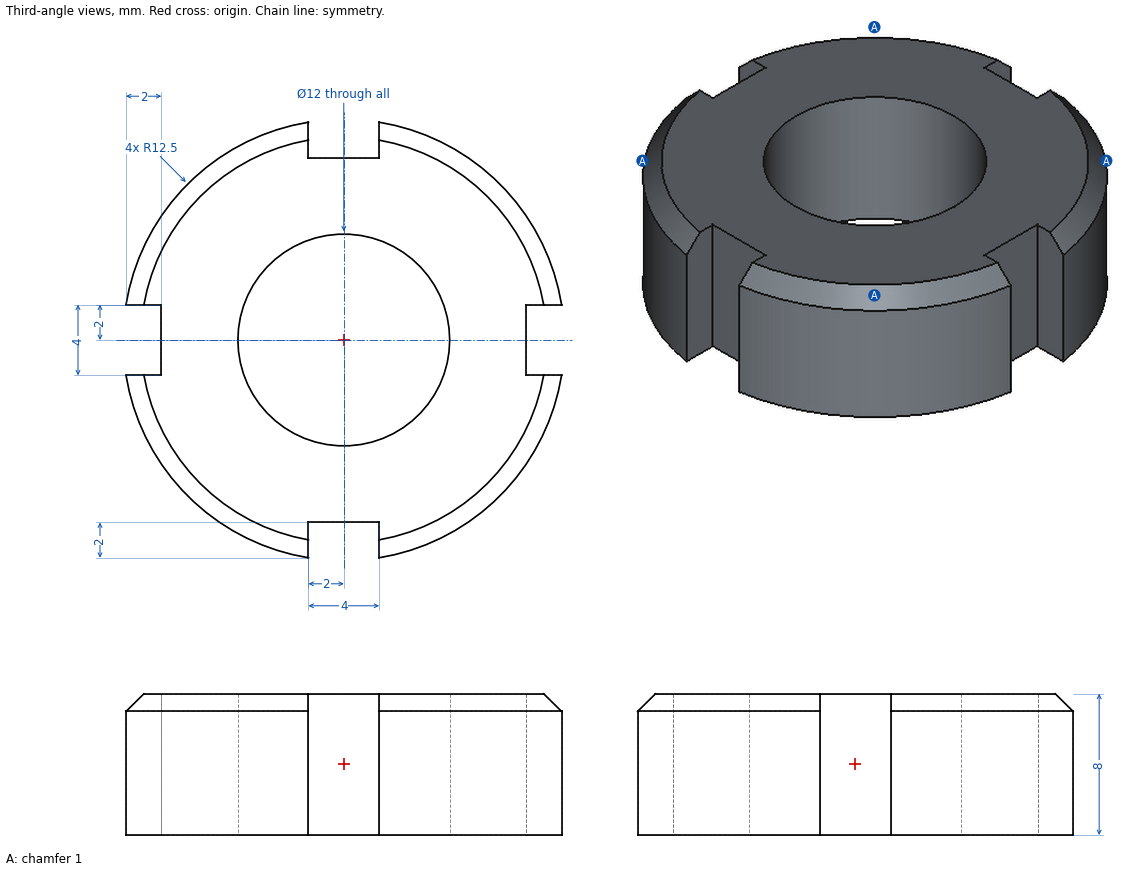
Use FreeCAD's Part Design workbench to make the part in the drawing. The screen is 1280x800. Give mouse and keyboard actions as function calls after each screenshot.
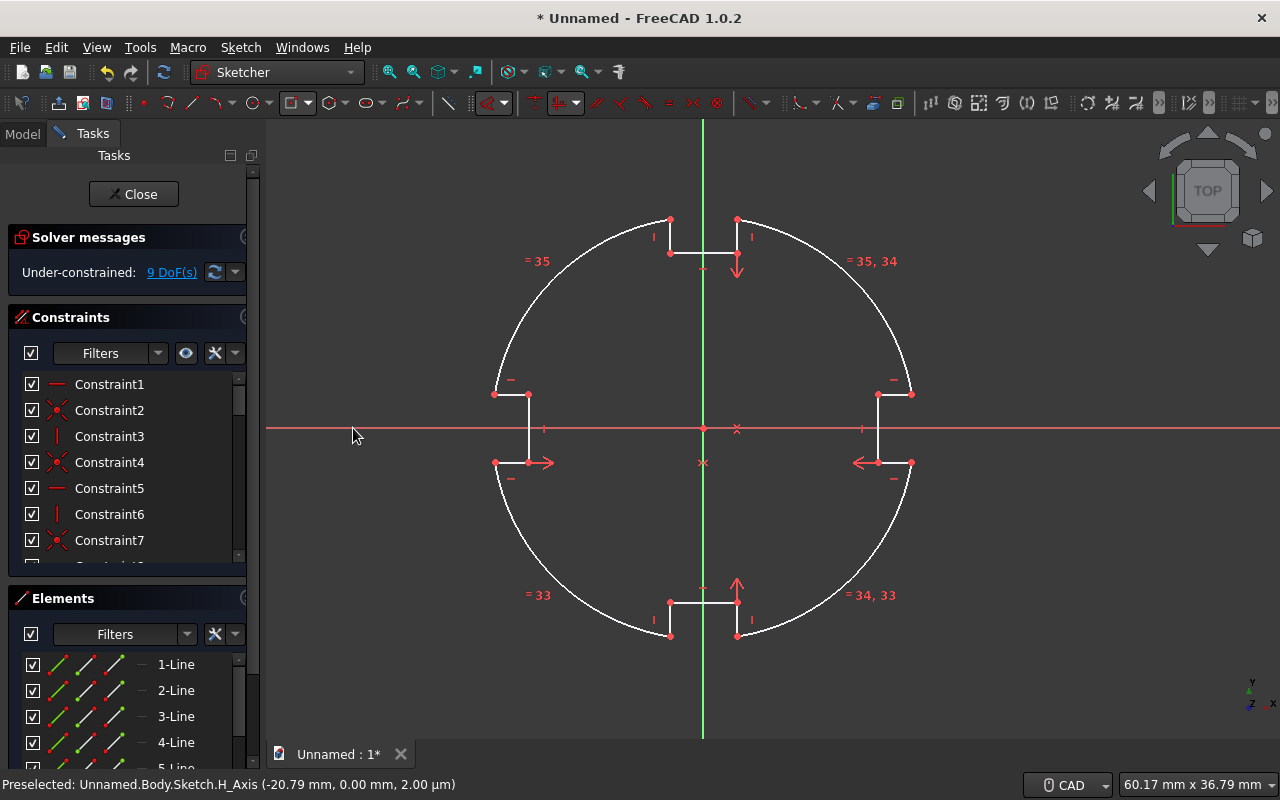
click(522, 537)
click(495, 553)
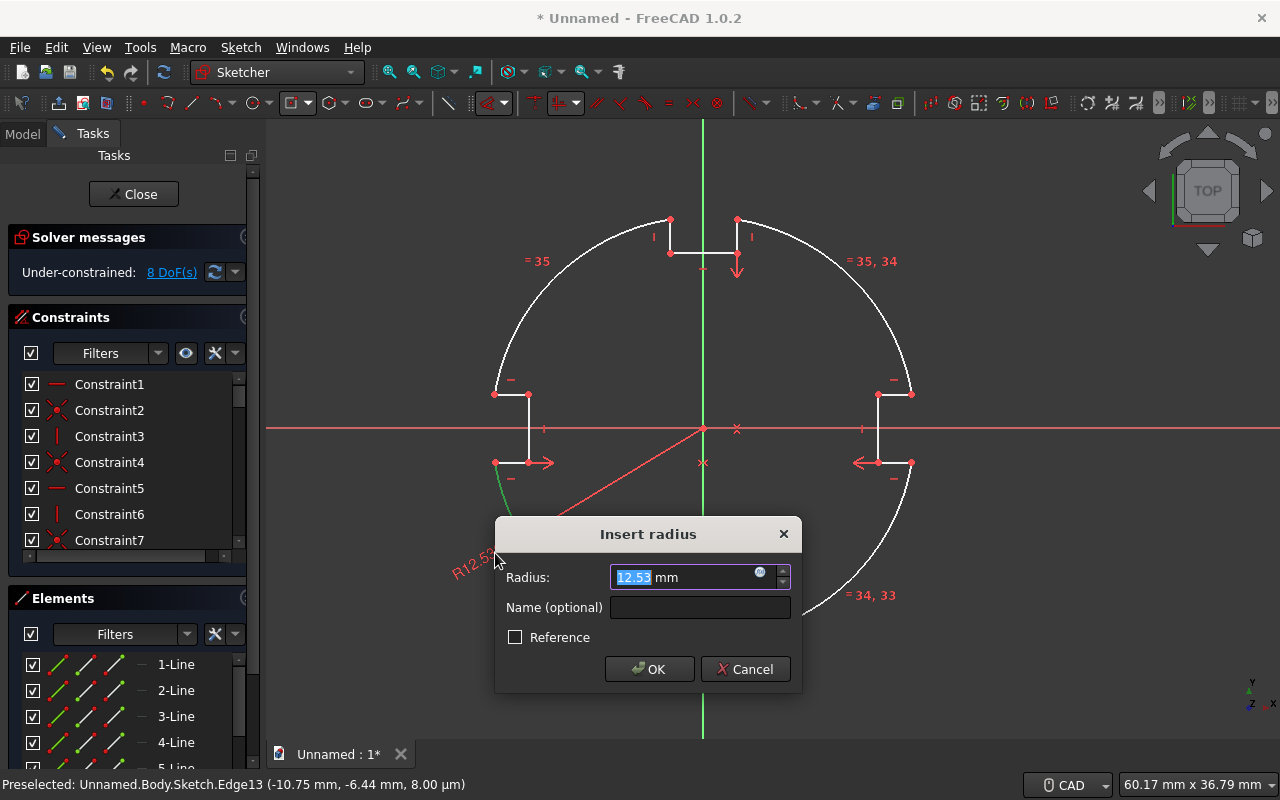
text(12.5)
key(Return)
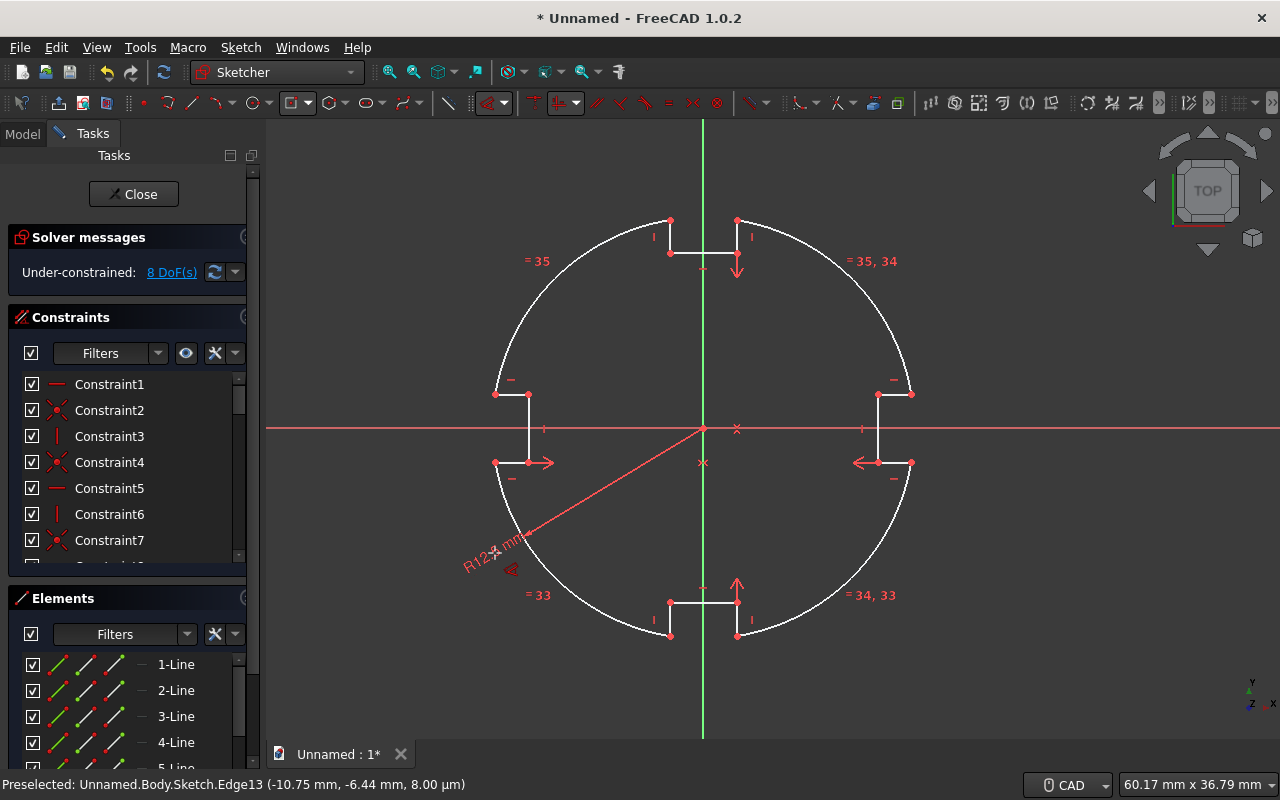
scroll(505, 395, up, 2)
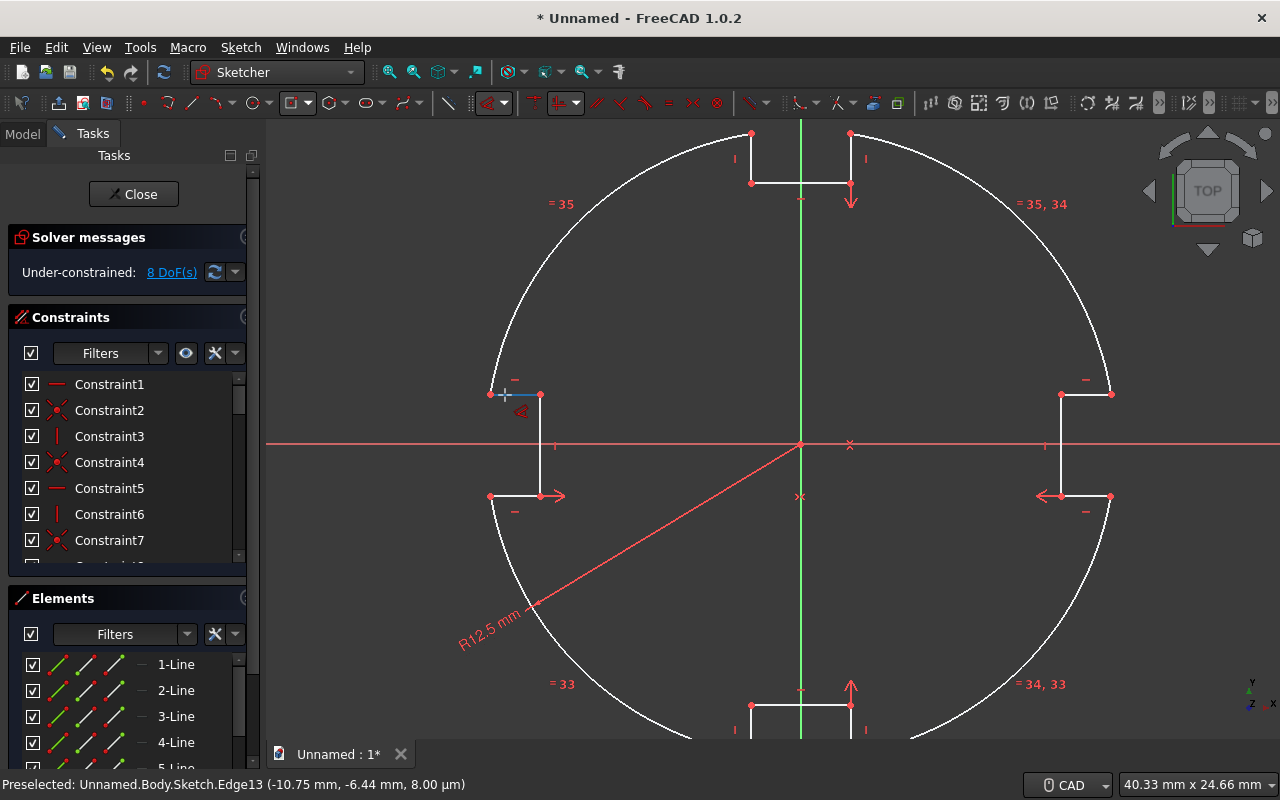
click(505, 395)
click(515, 361)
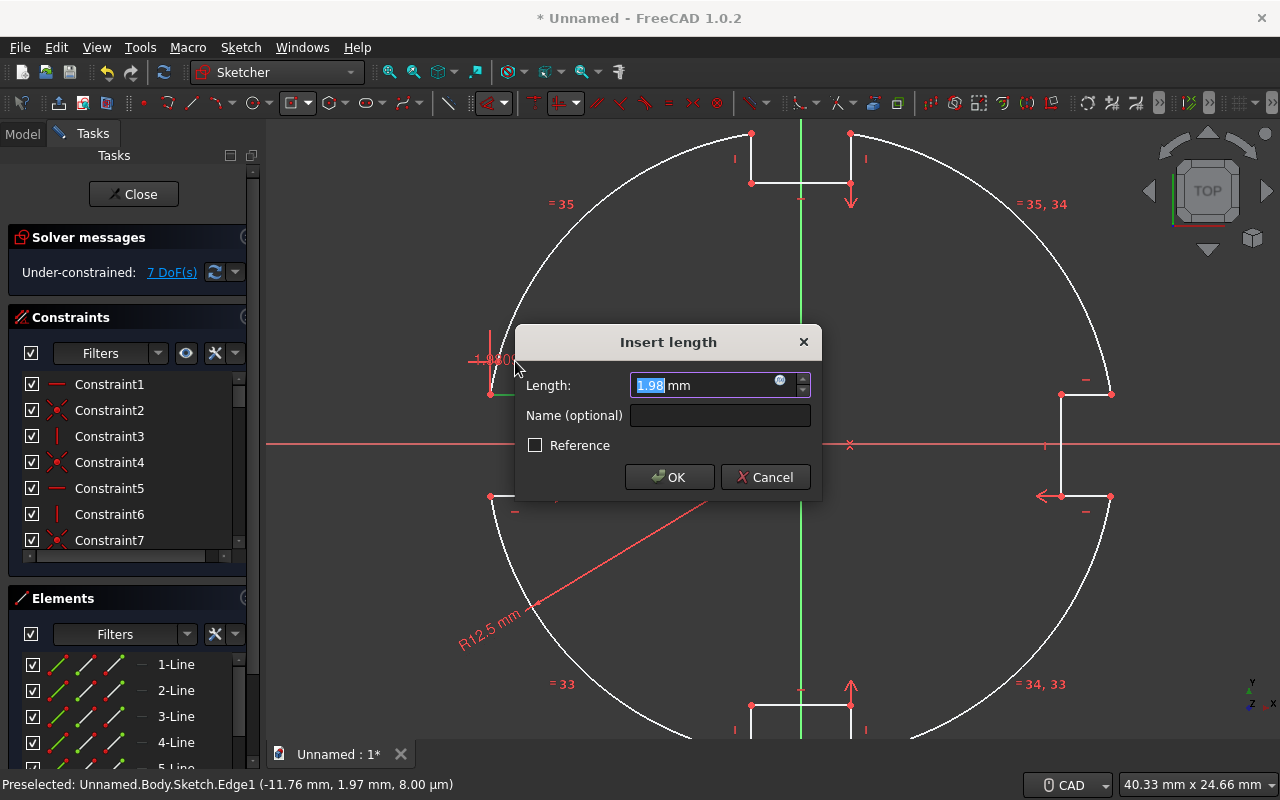
text(2)
key(Return)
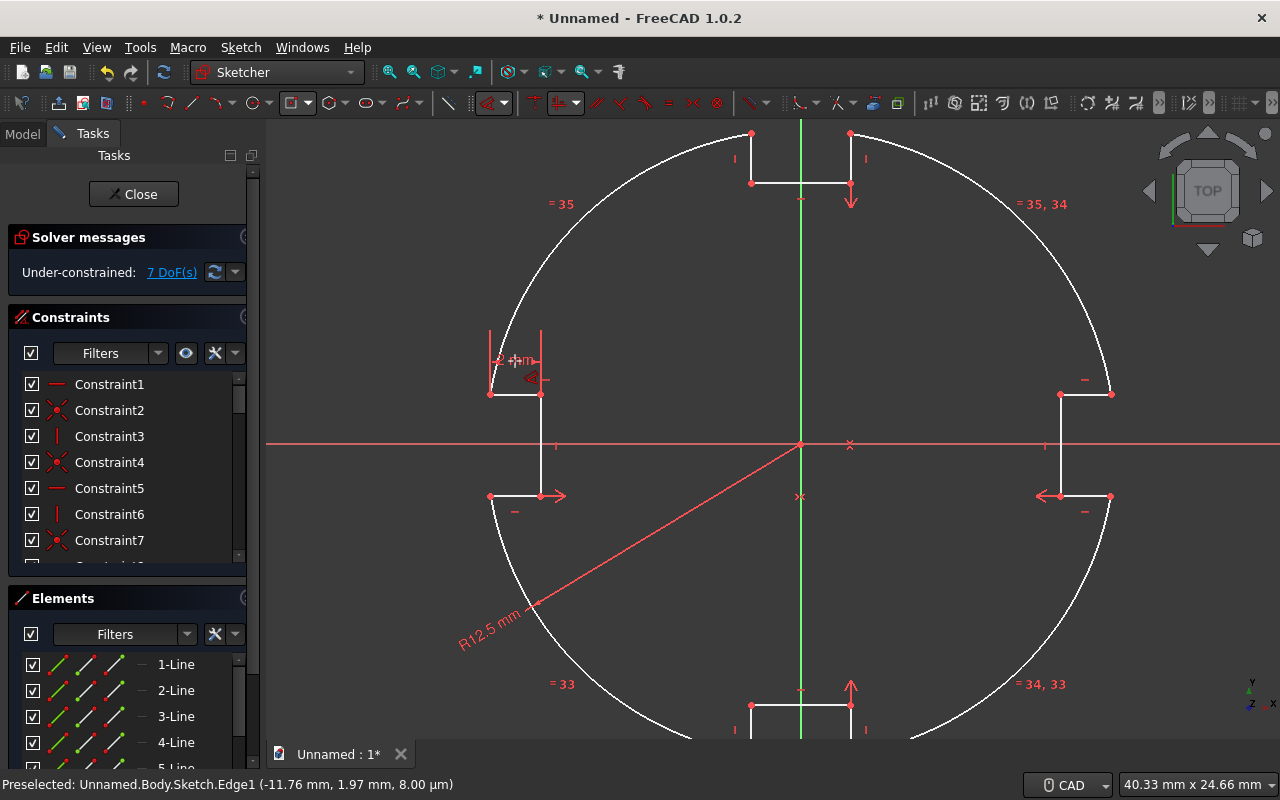
click(541, 425)
click(507, 422)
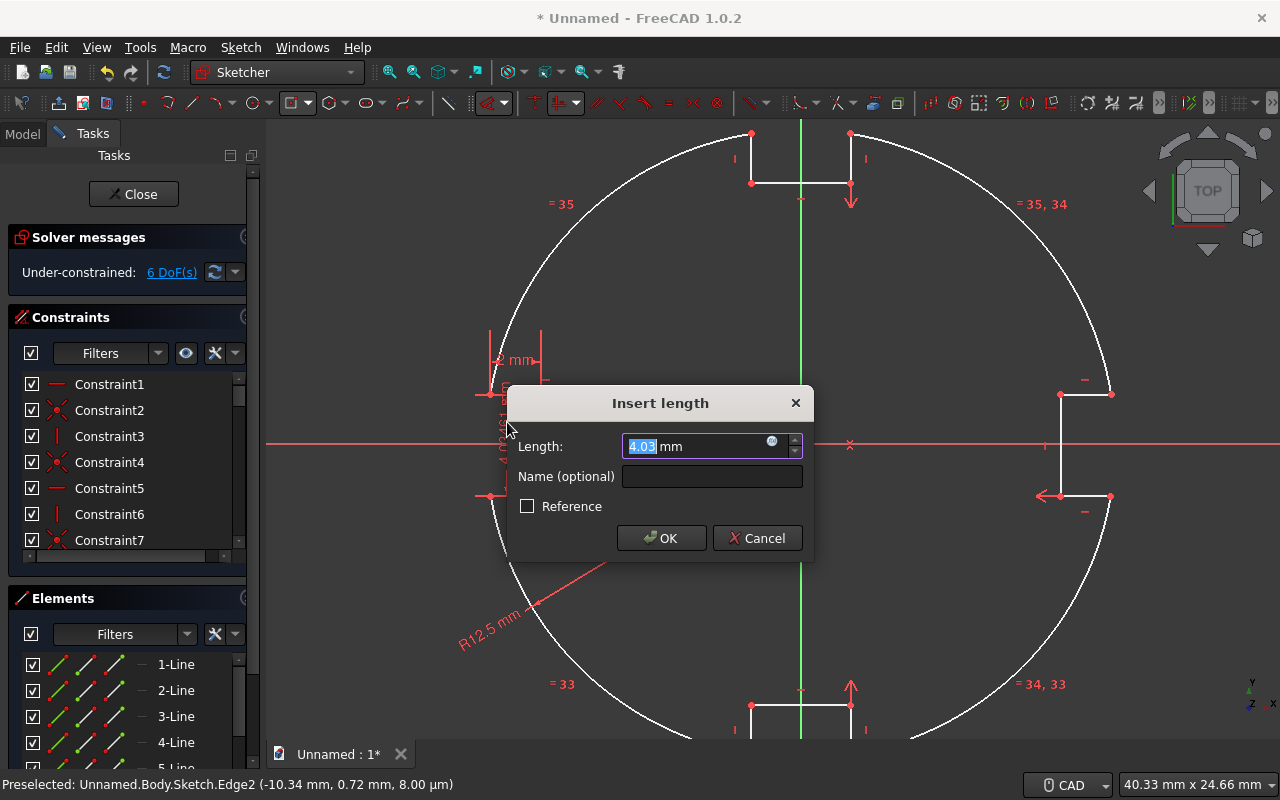
text(4)
key(Return)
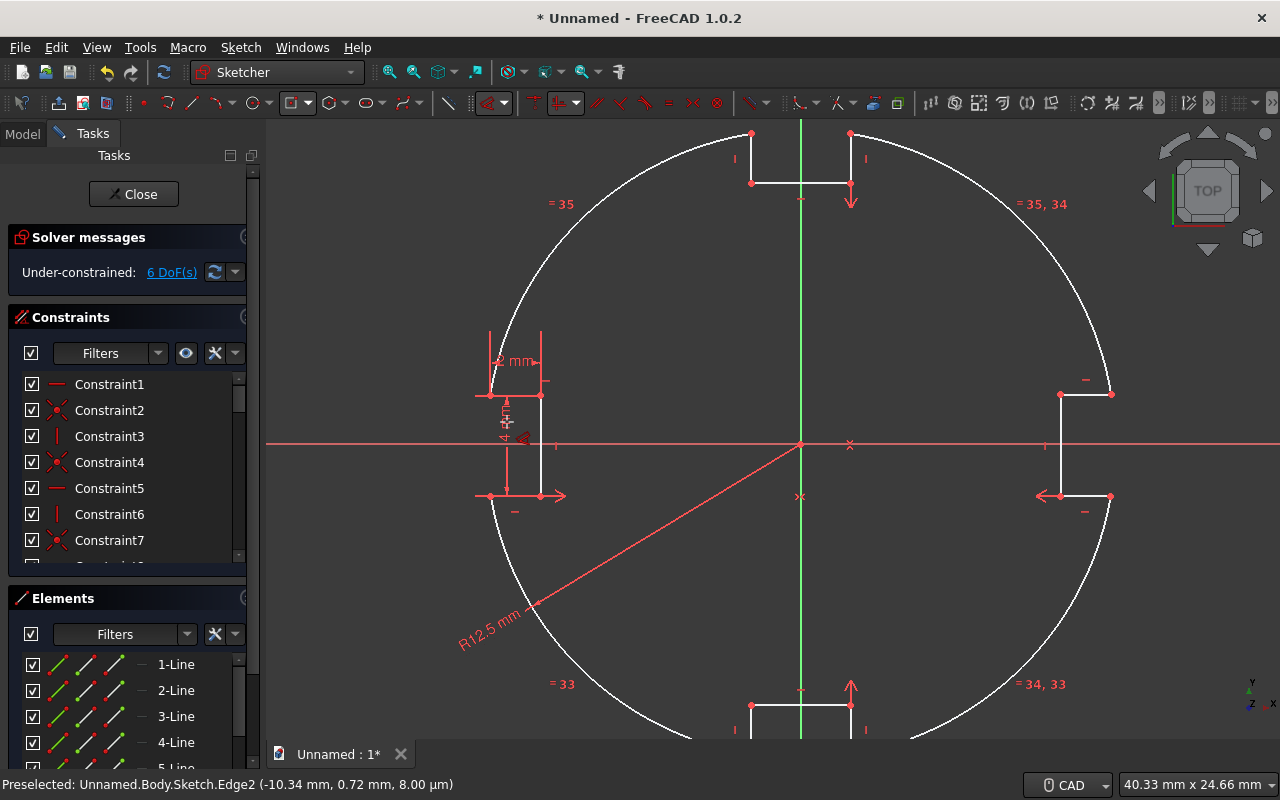
scroll(509, 398, down, 2)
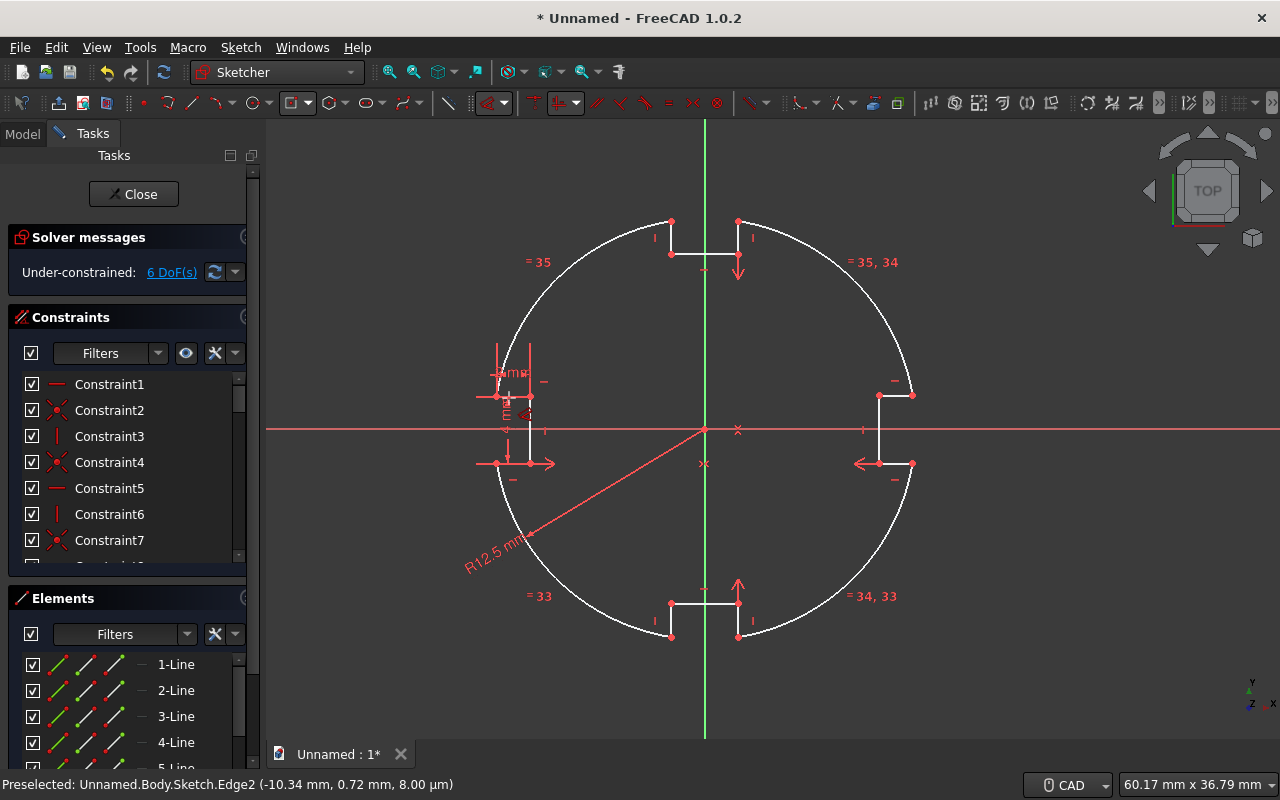
scroll(671, 627, up, 2)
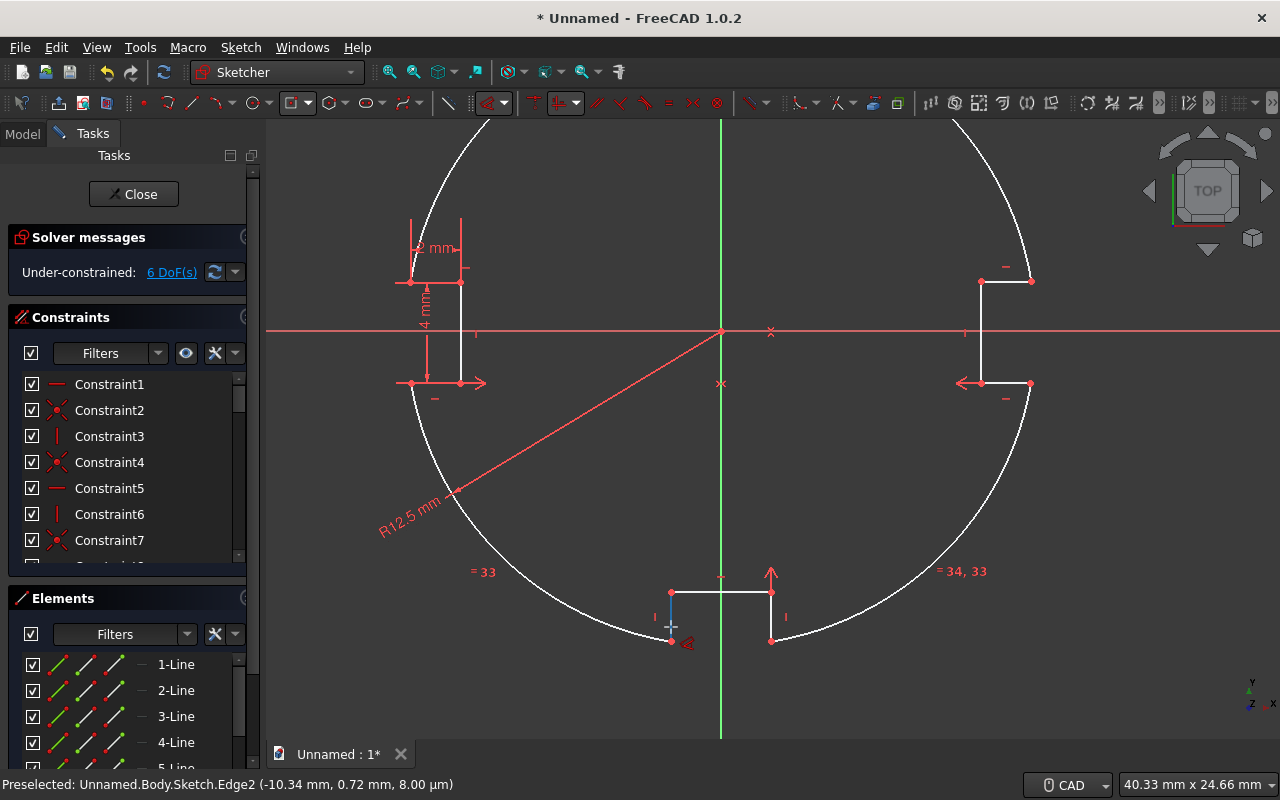
click(671, 627)
click(637, 617)